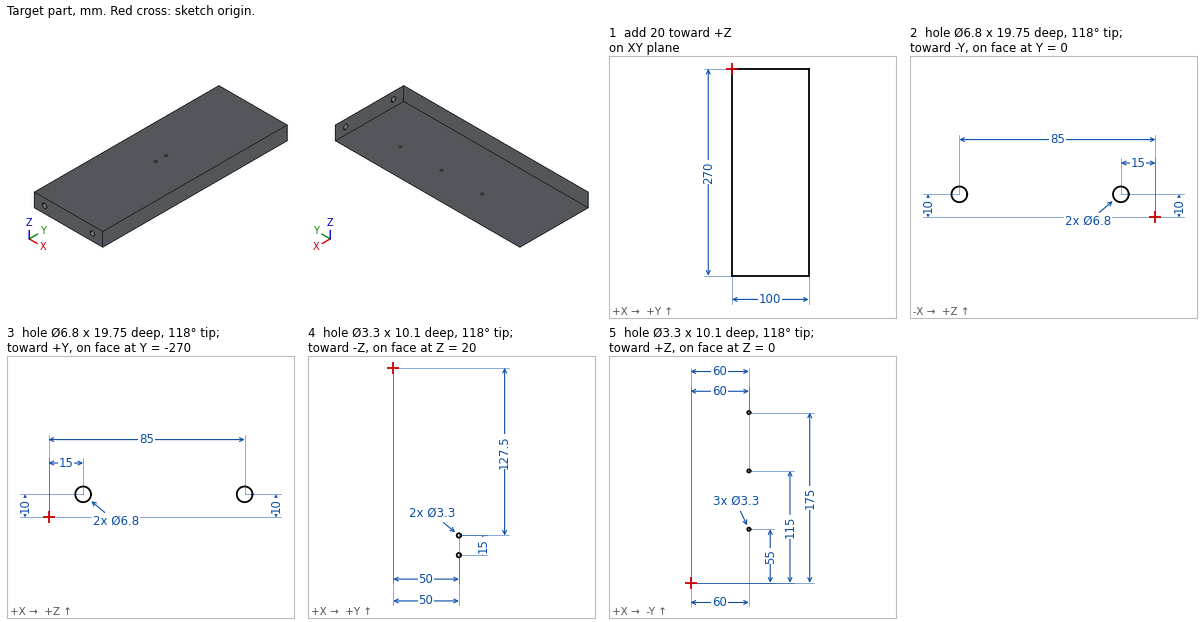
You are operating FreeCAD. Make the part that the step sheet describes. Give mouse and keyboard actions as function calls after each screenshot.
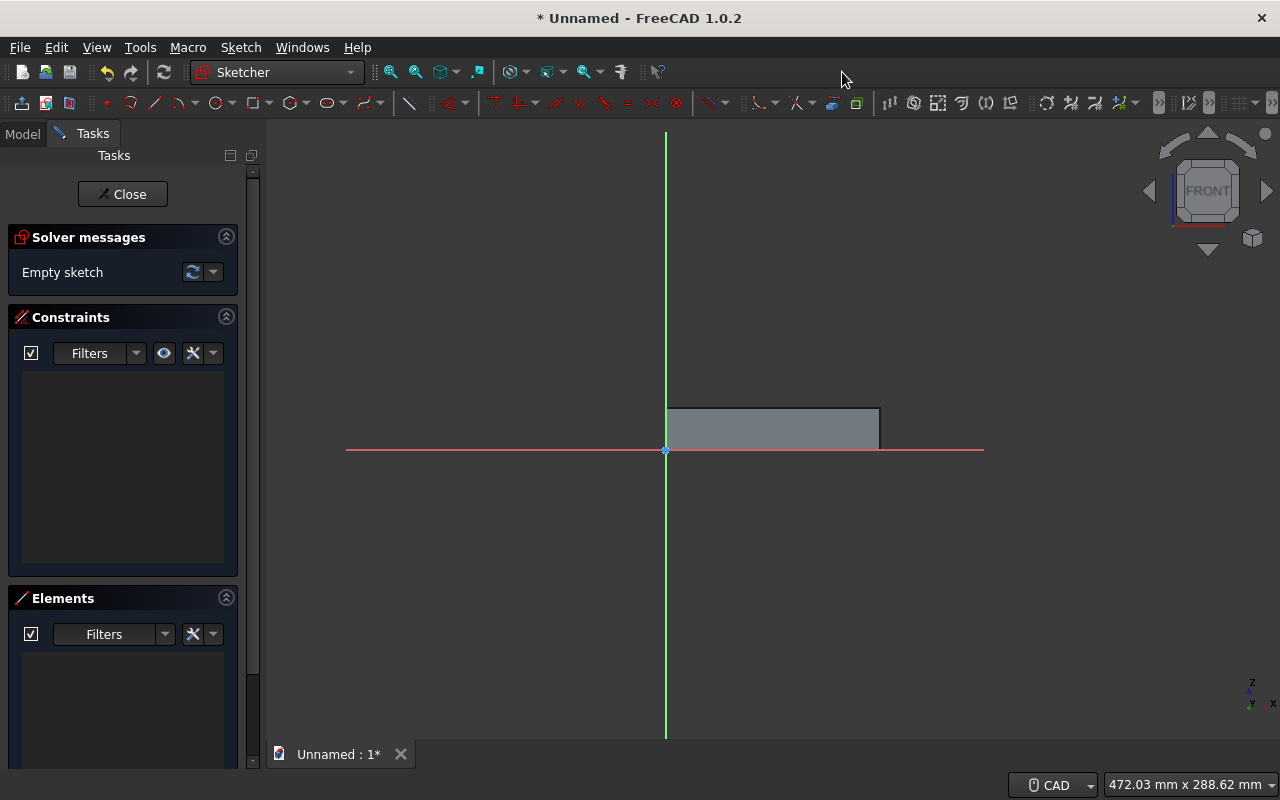
scroll(785, 439, up, 6)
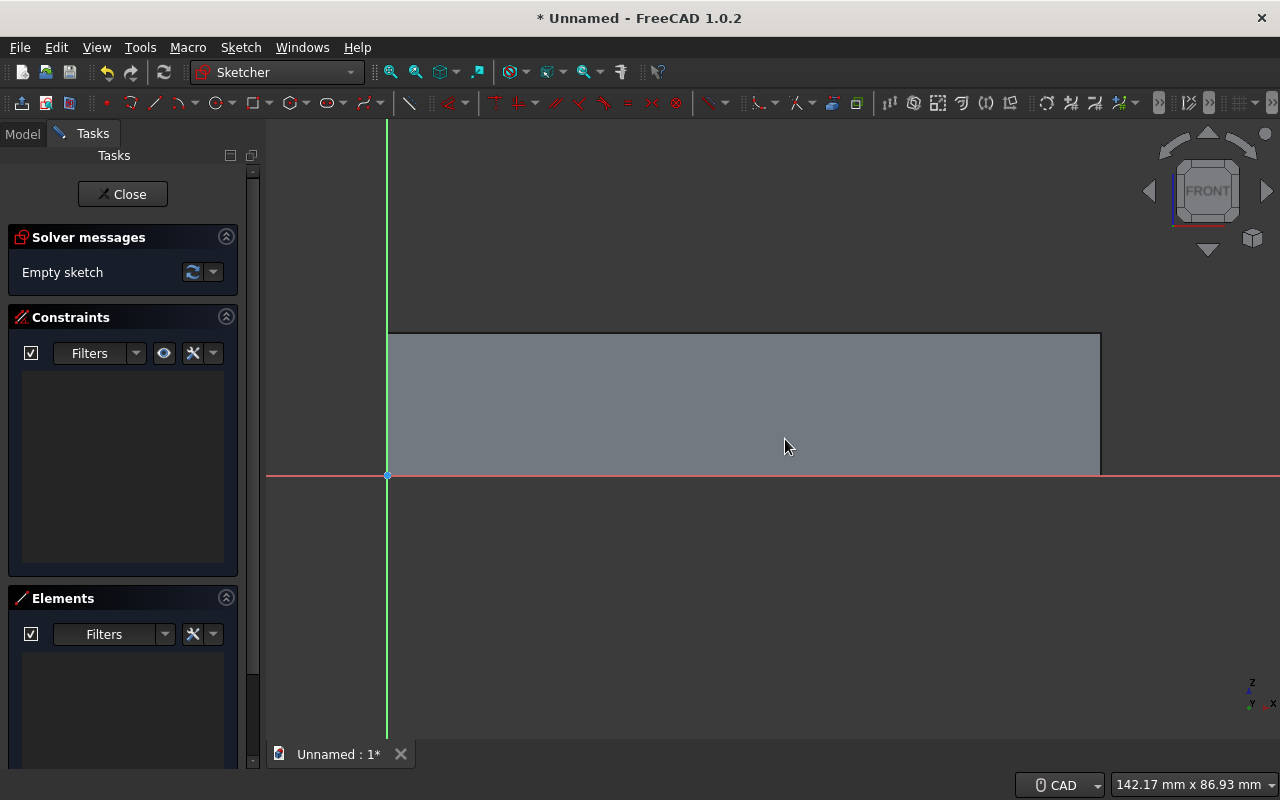
click(216, 104)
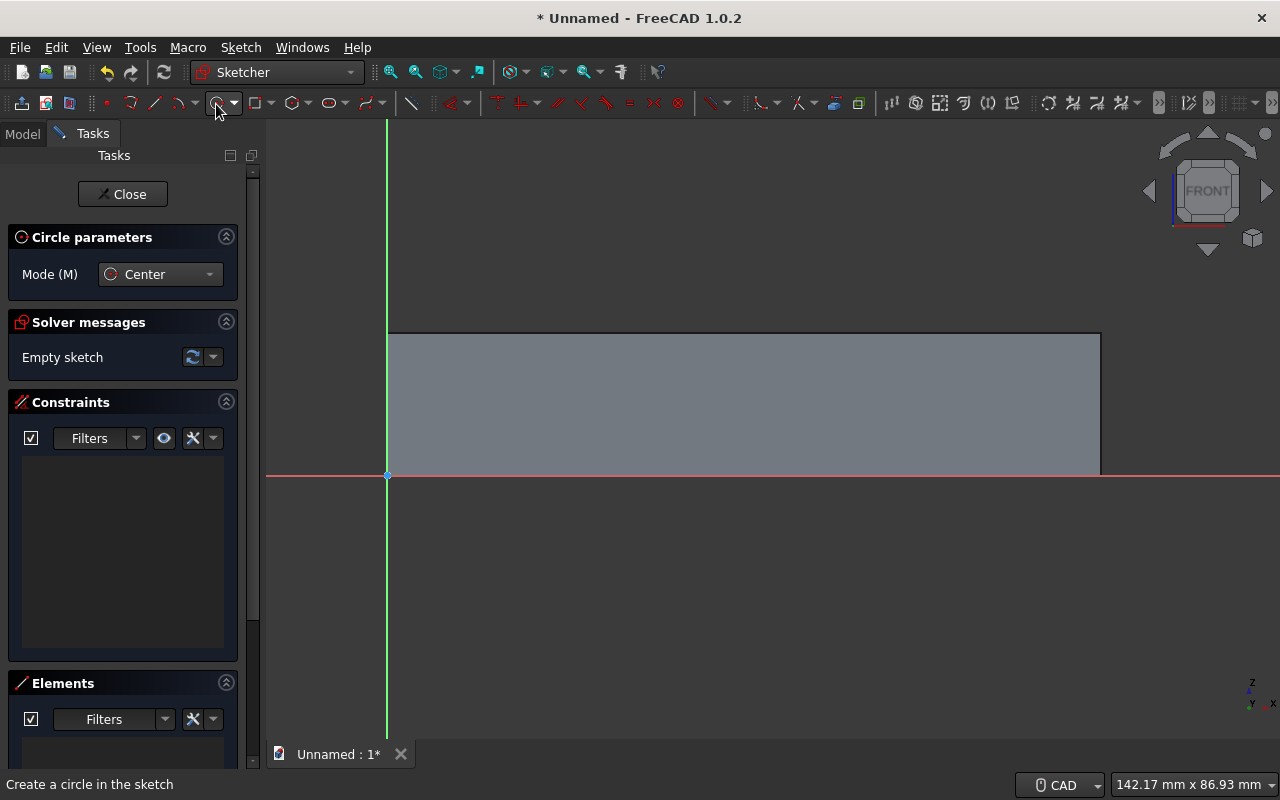
click(494, 405)
click(511, 387)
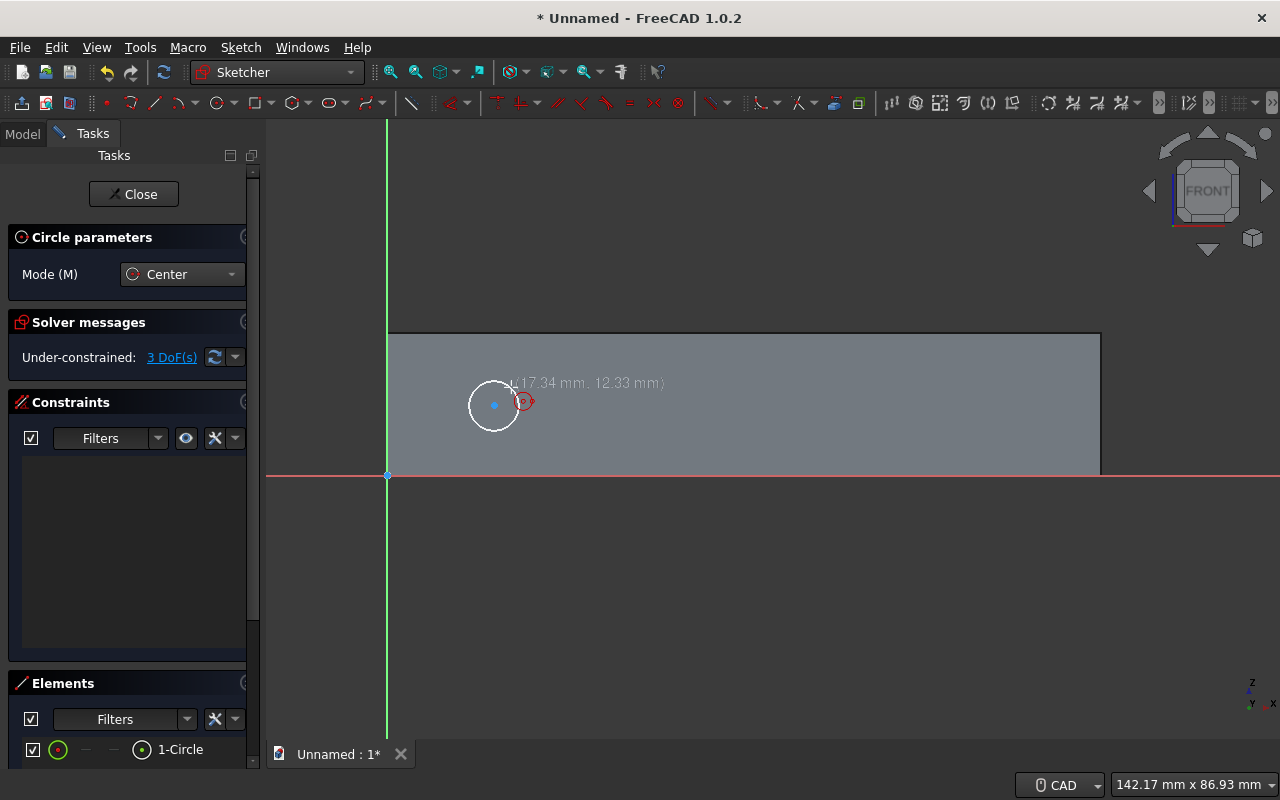
click(994, 405)
click(1011, 387)
key(Escape)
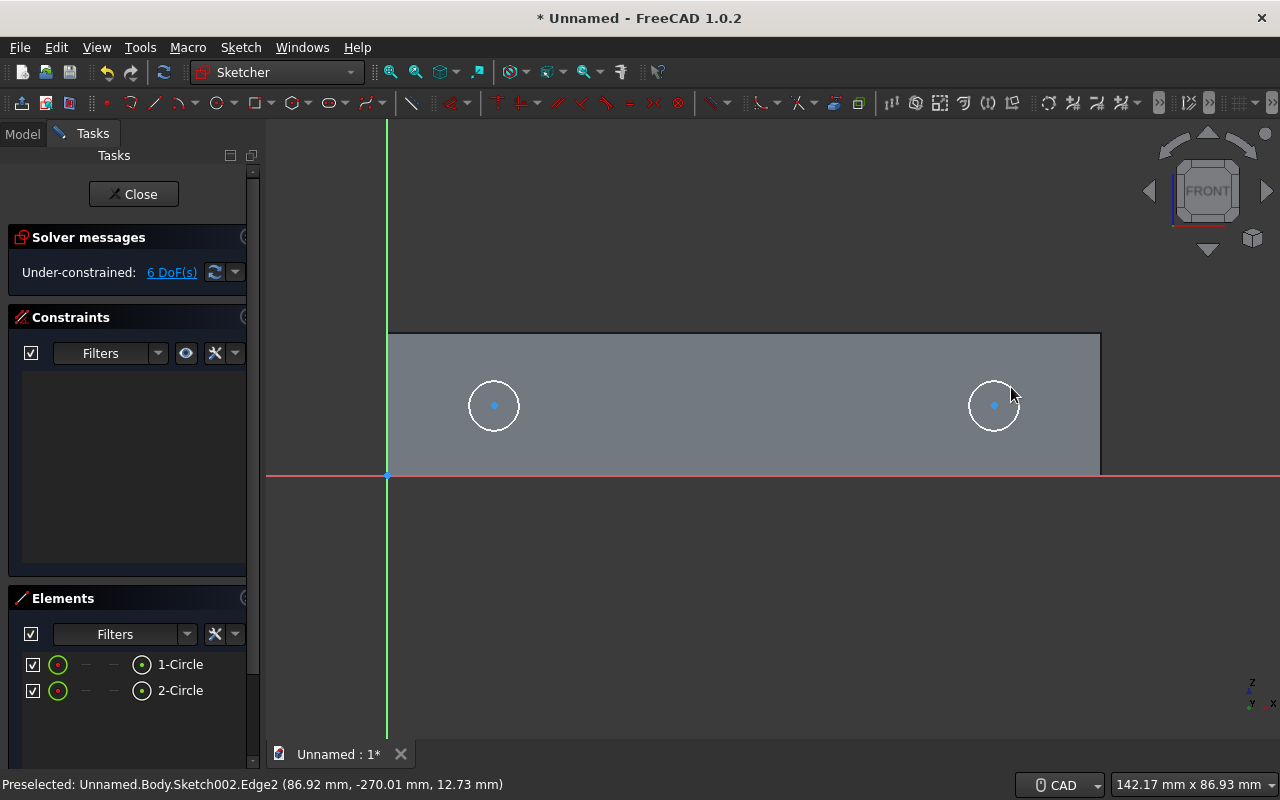
click(511, 388)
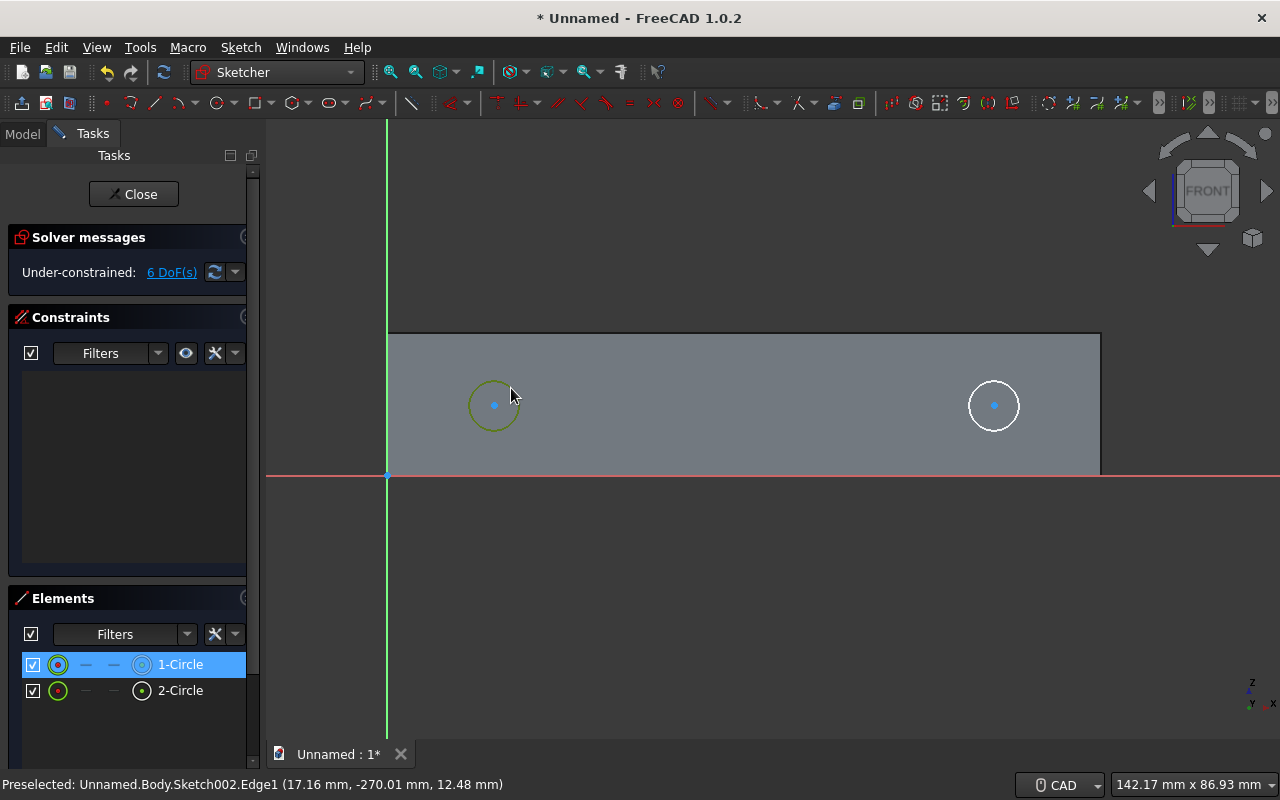
click(1011, 388)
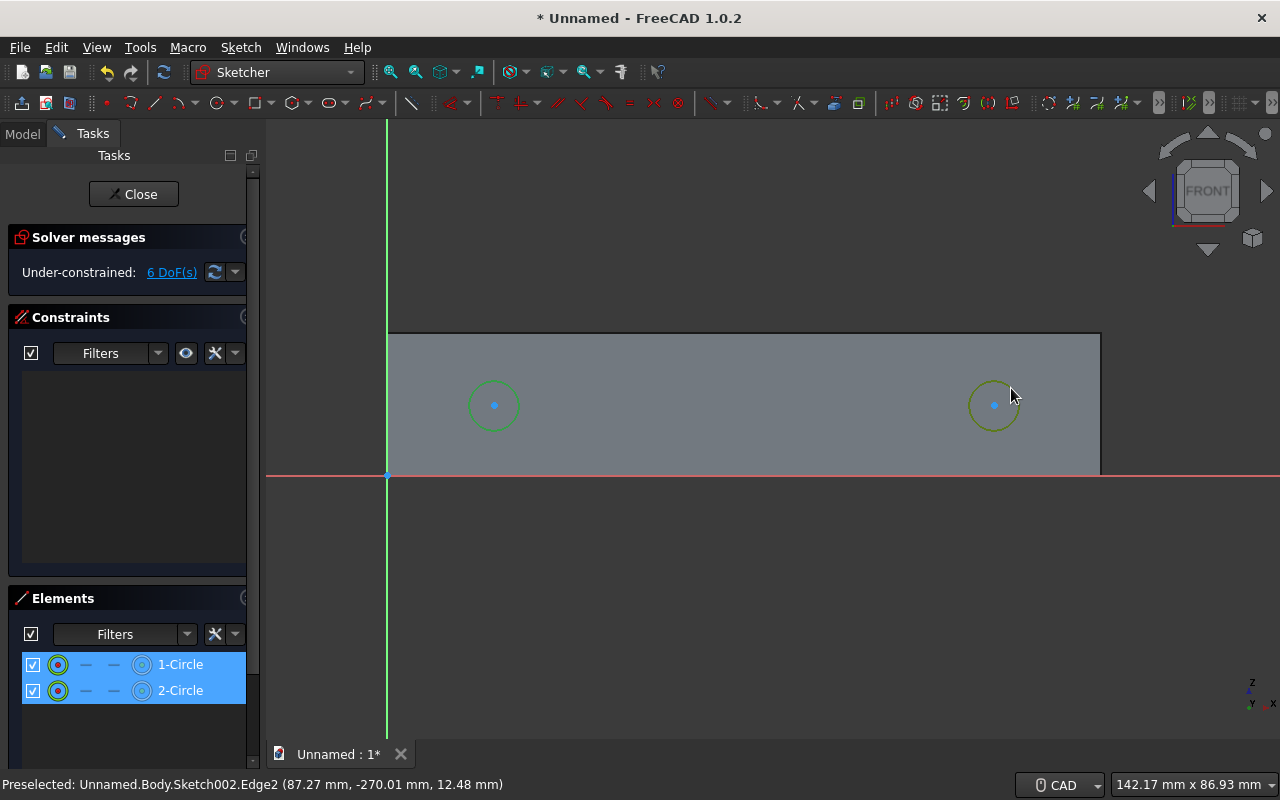
click(630, 104)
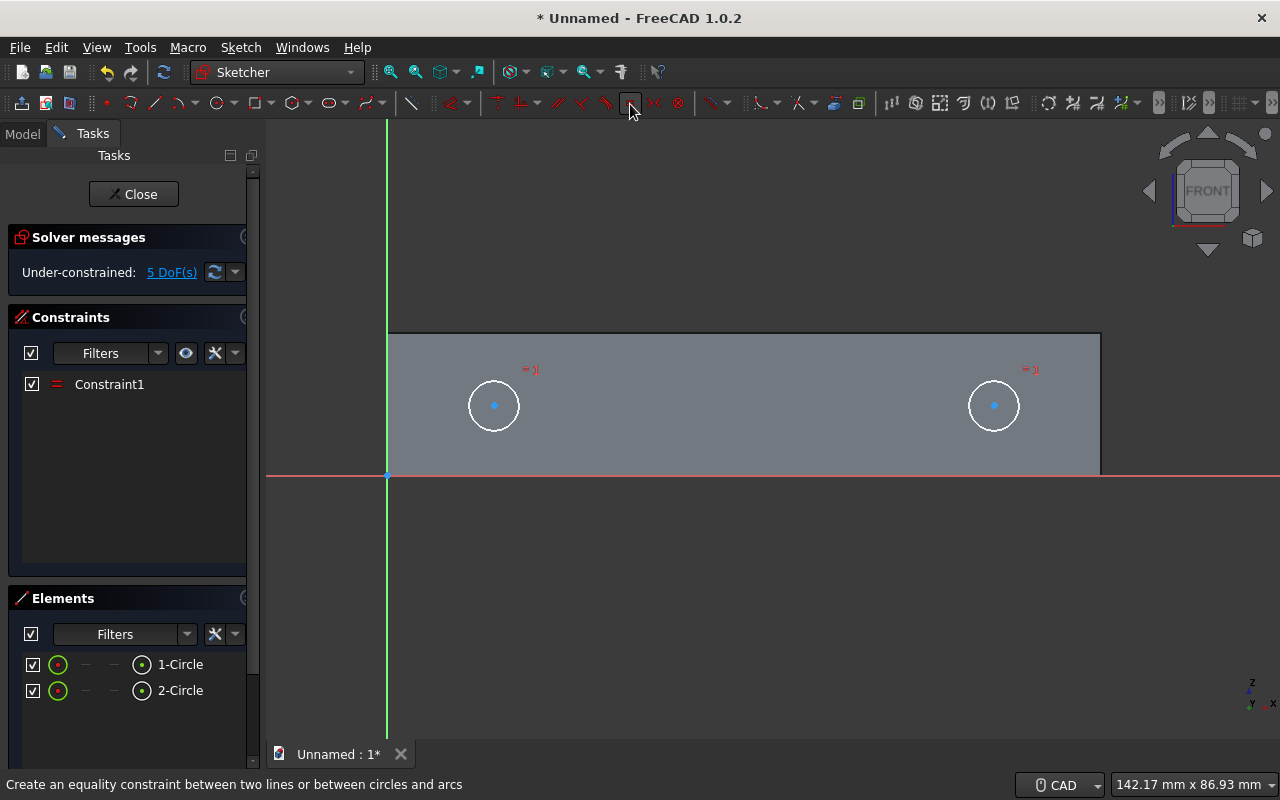
click(450, 104)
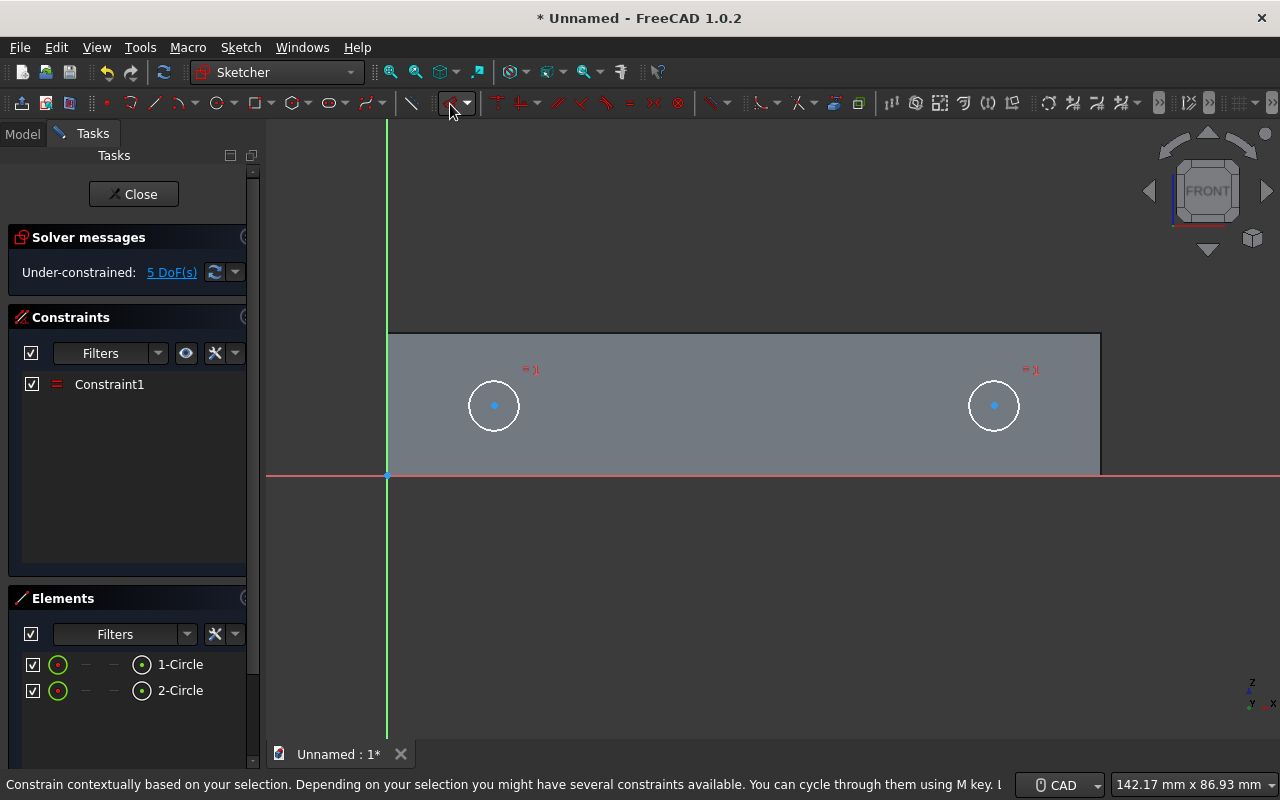
click(511, 388)
click(533, 365)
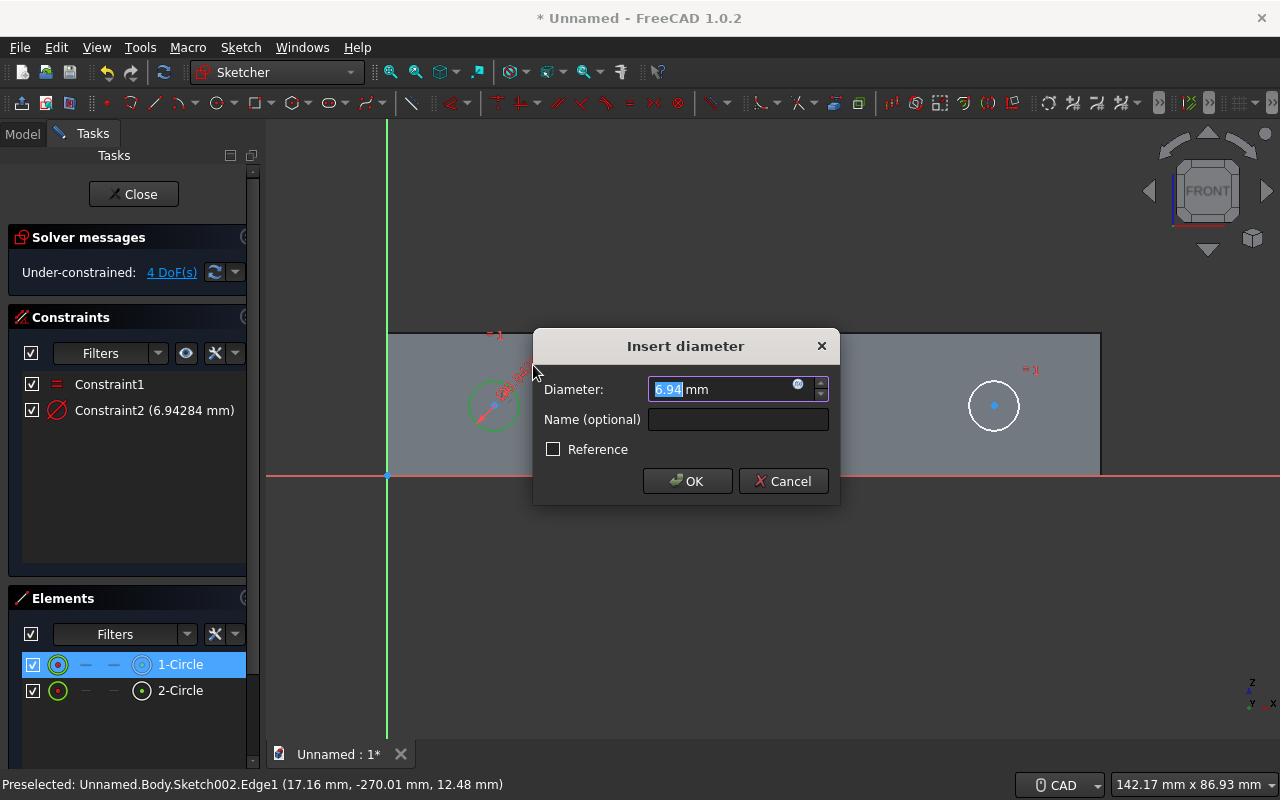
text(6.8)
key(Return)